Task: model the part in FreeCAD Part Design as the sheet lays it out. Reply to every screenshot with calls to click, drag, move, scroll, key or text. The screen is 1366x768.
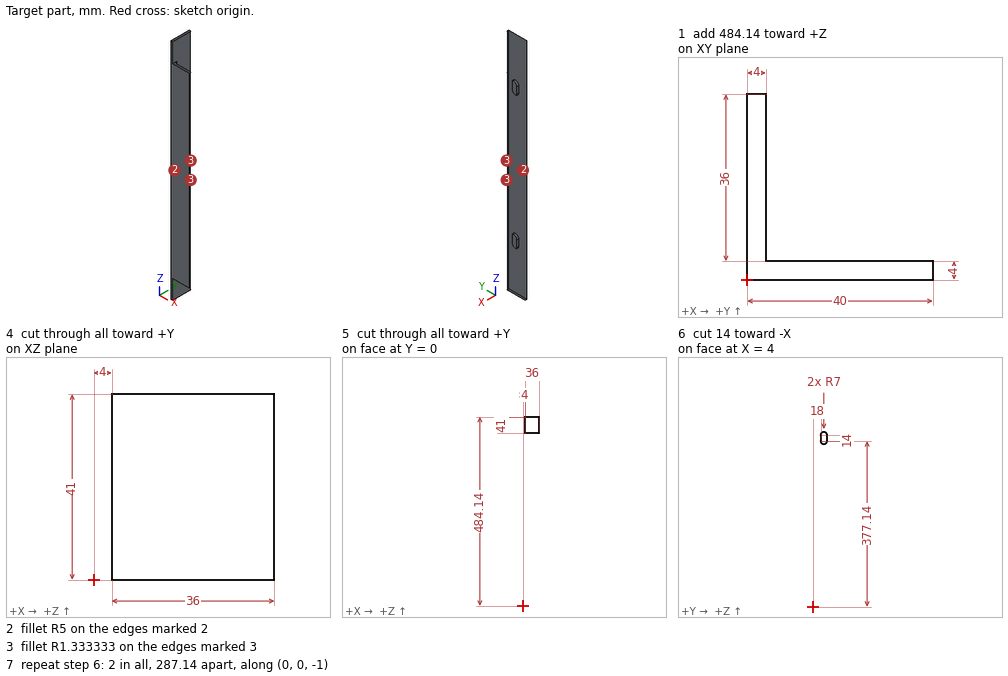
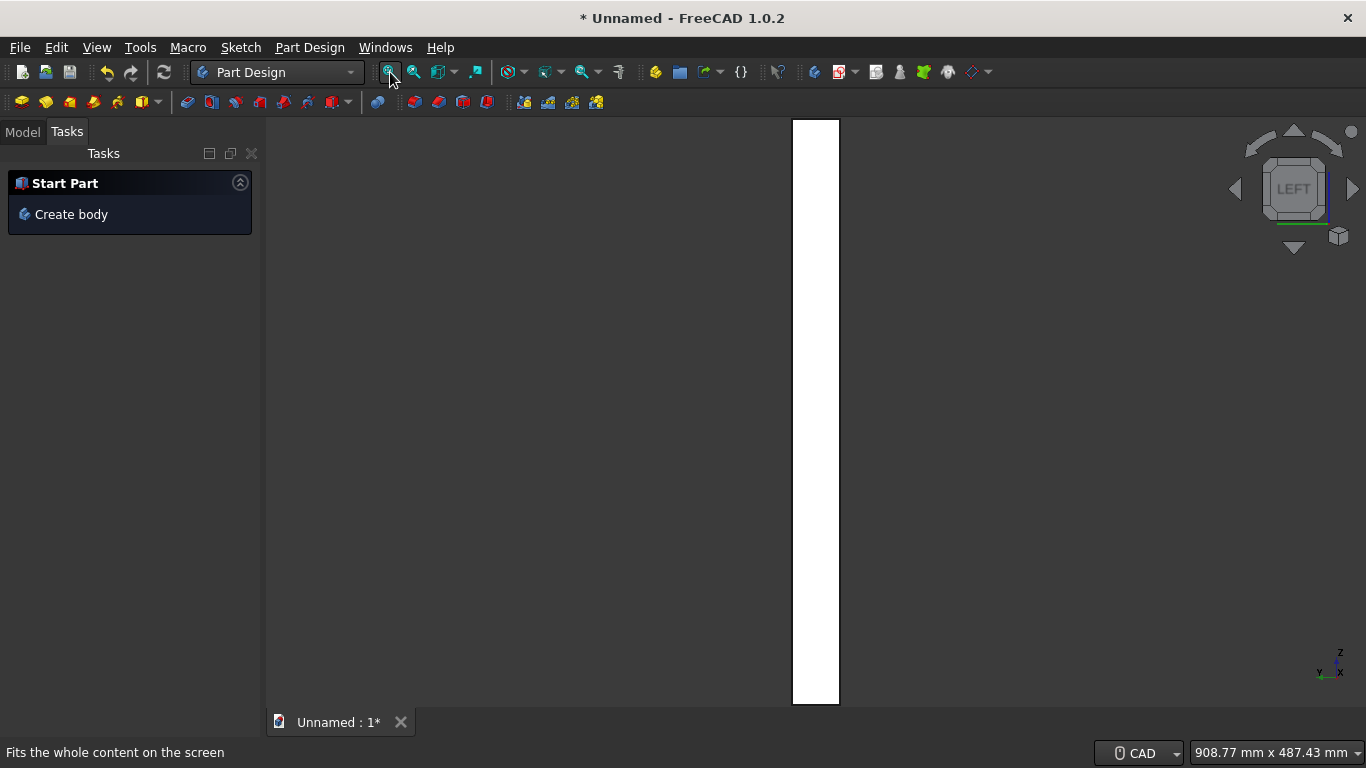
key(v)
key(3)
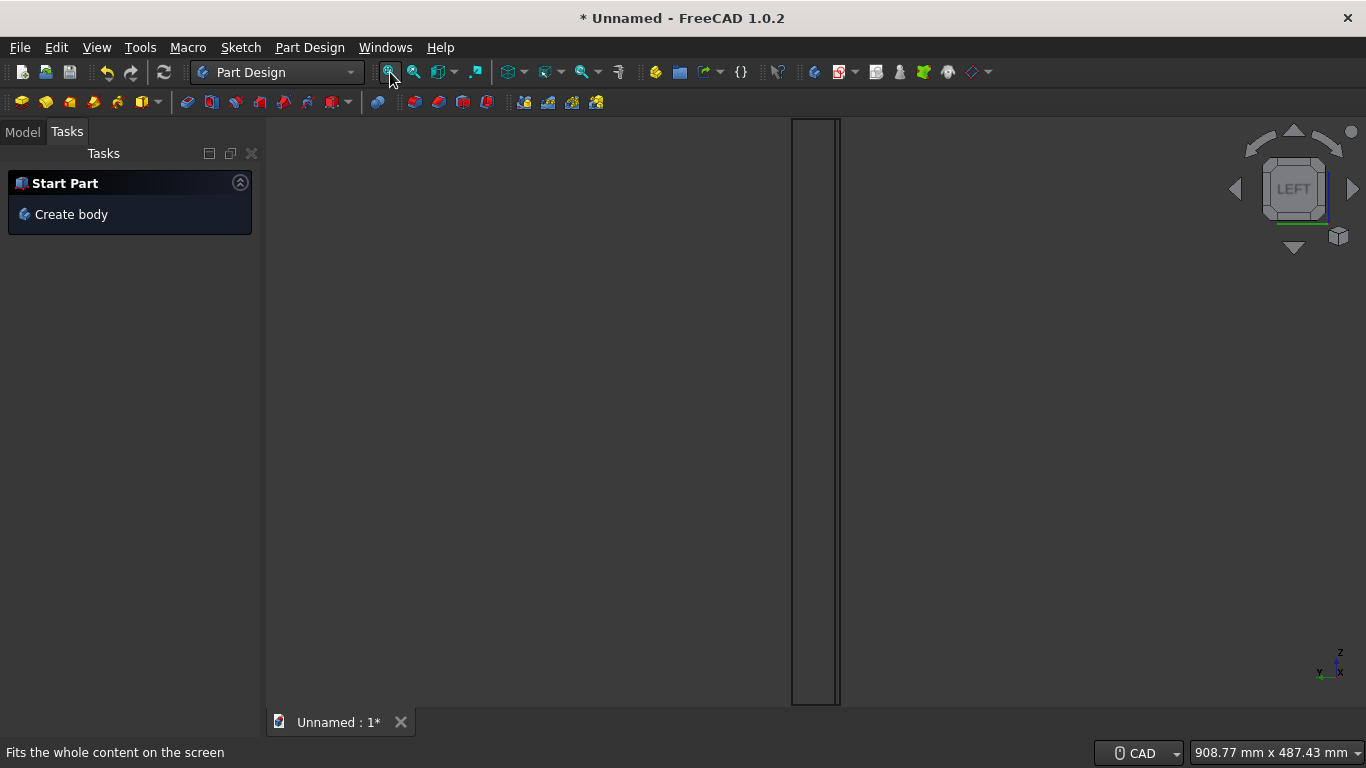
key(0)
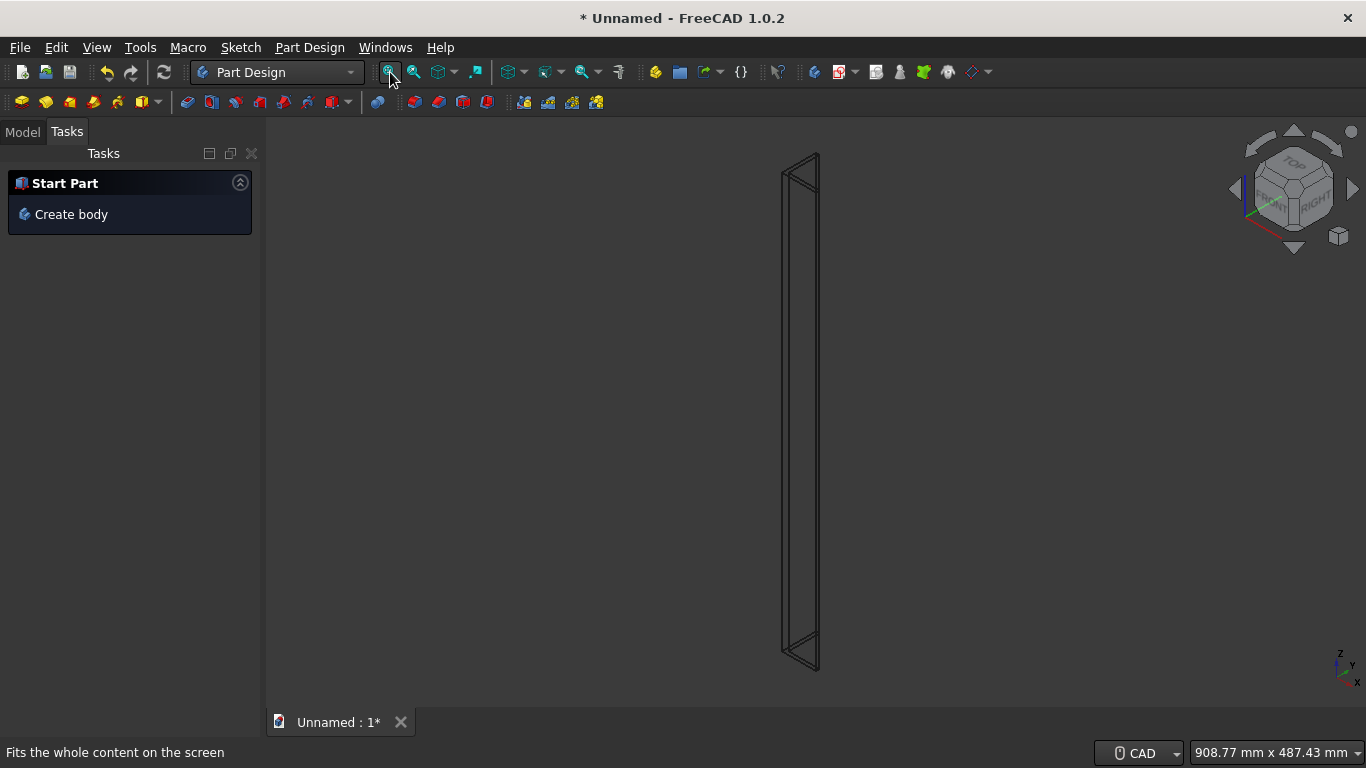
click(789, 411)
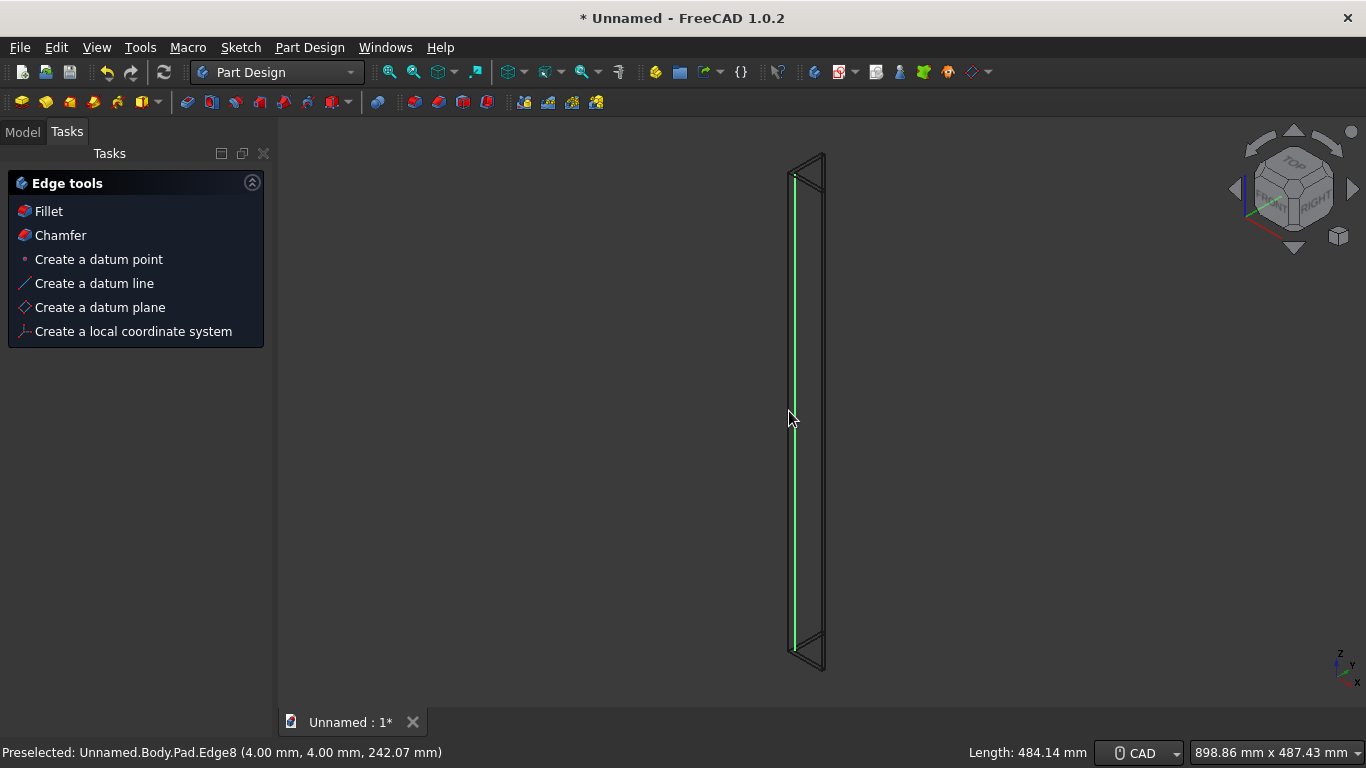
key(v)
key(1)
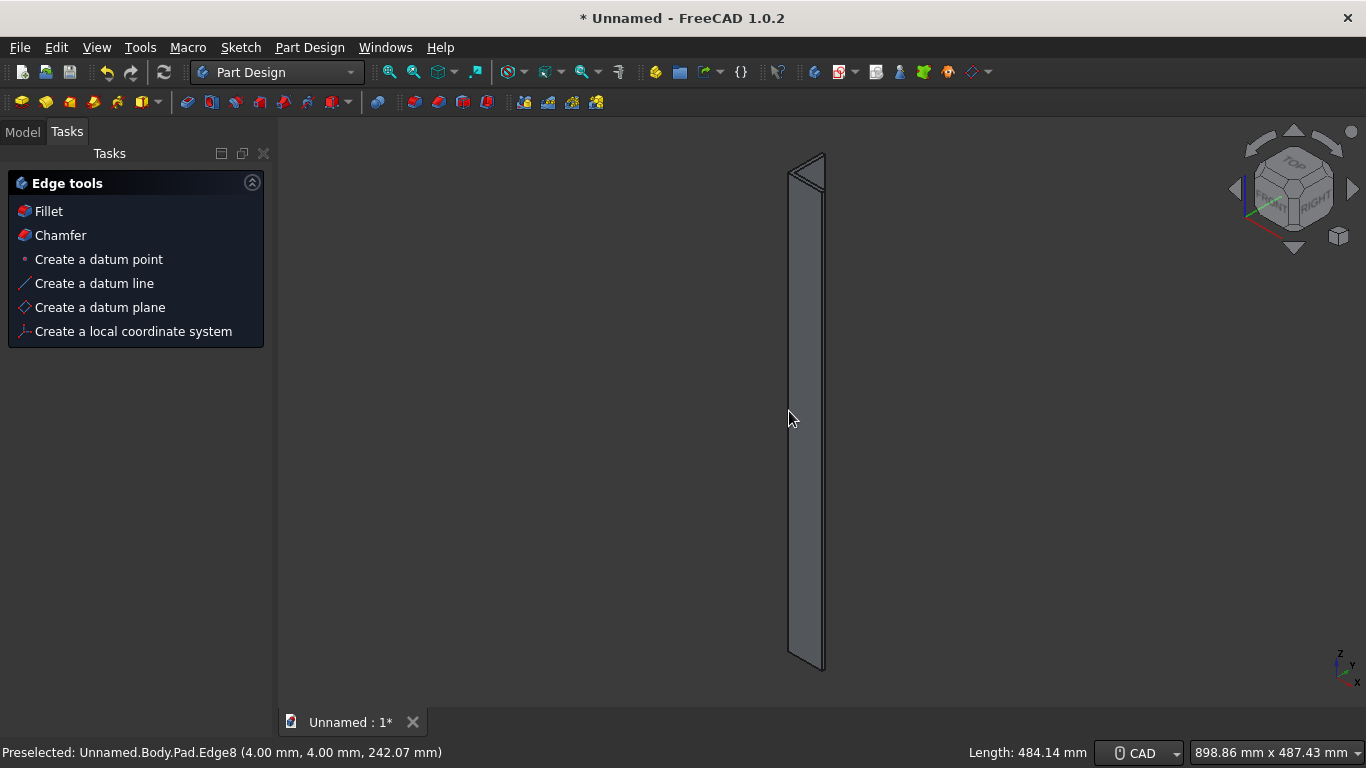
click(416, 102)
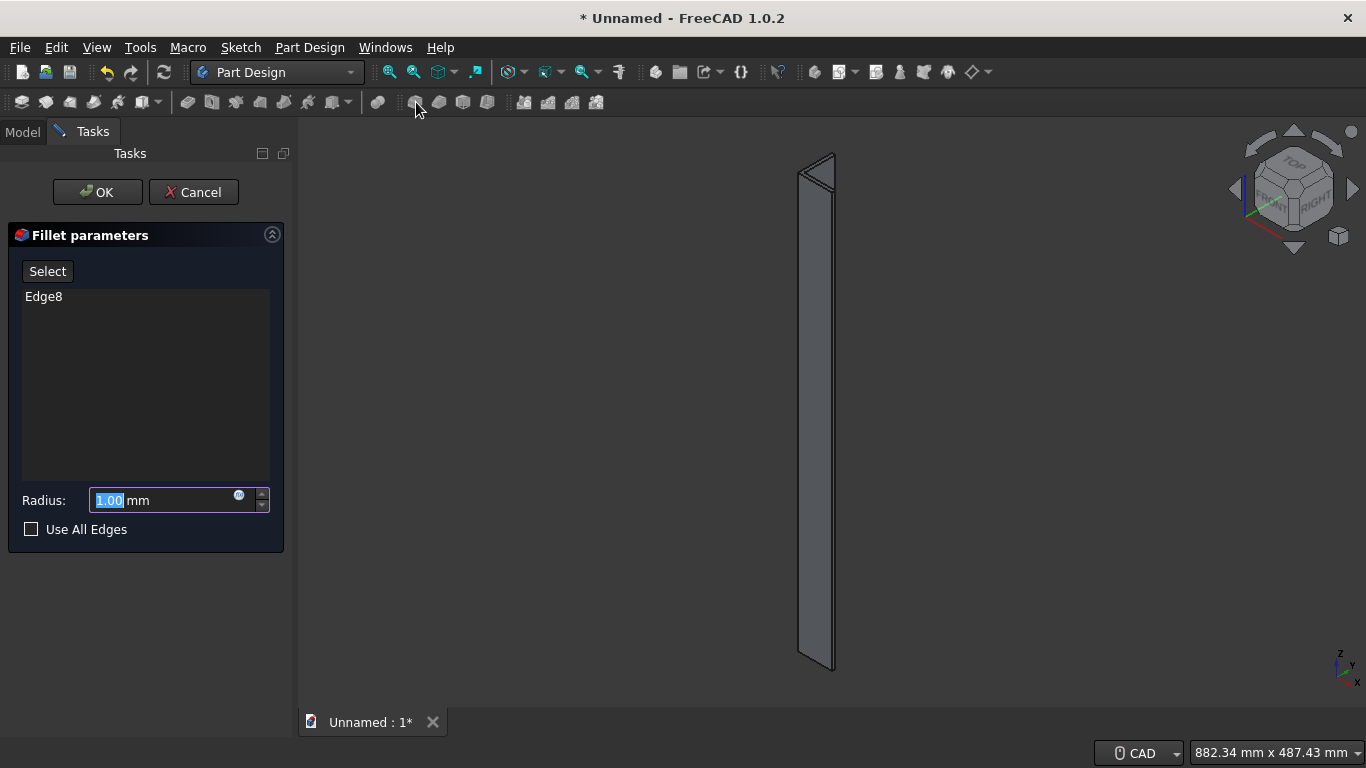
text(5)
key(Tab)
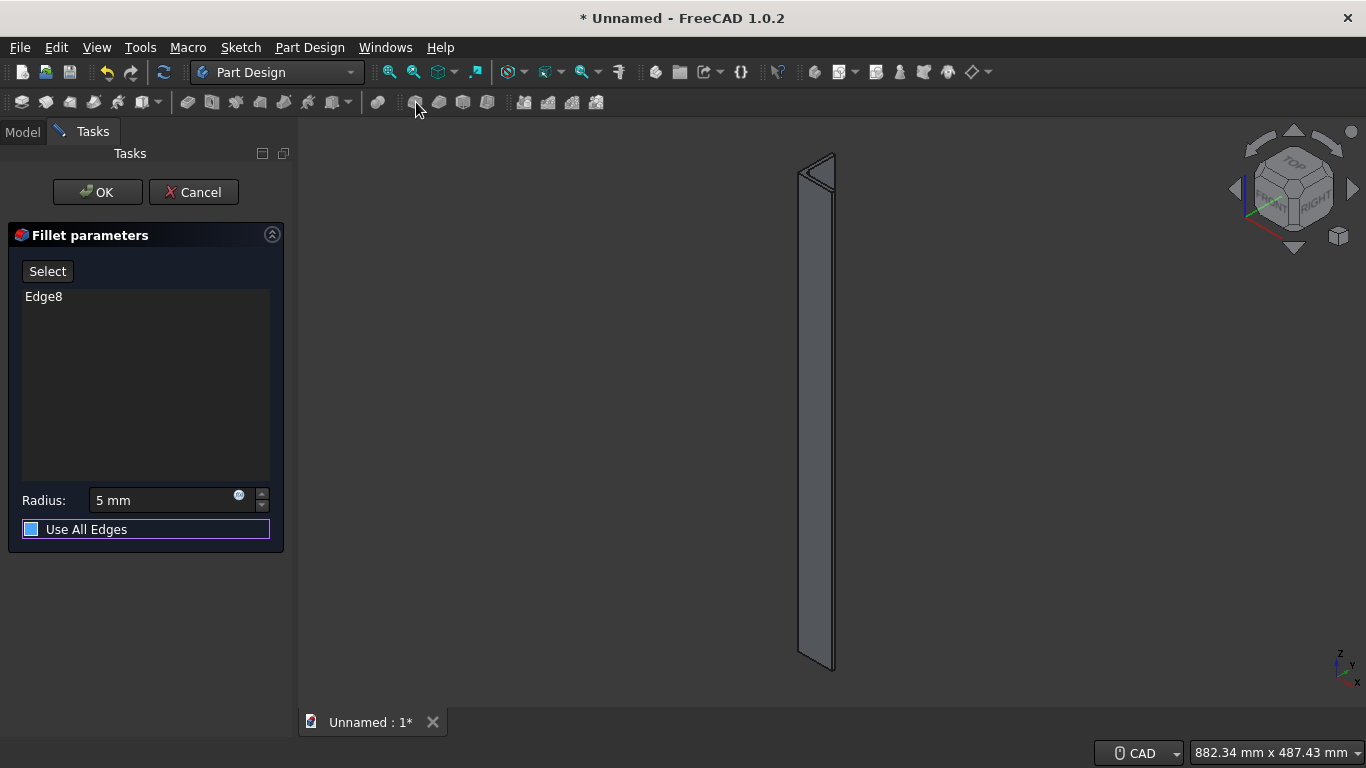
click(98, 192)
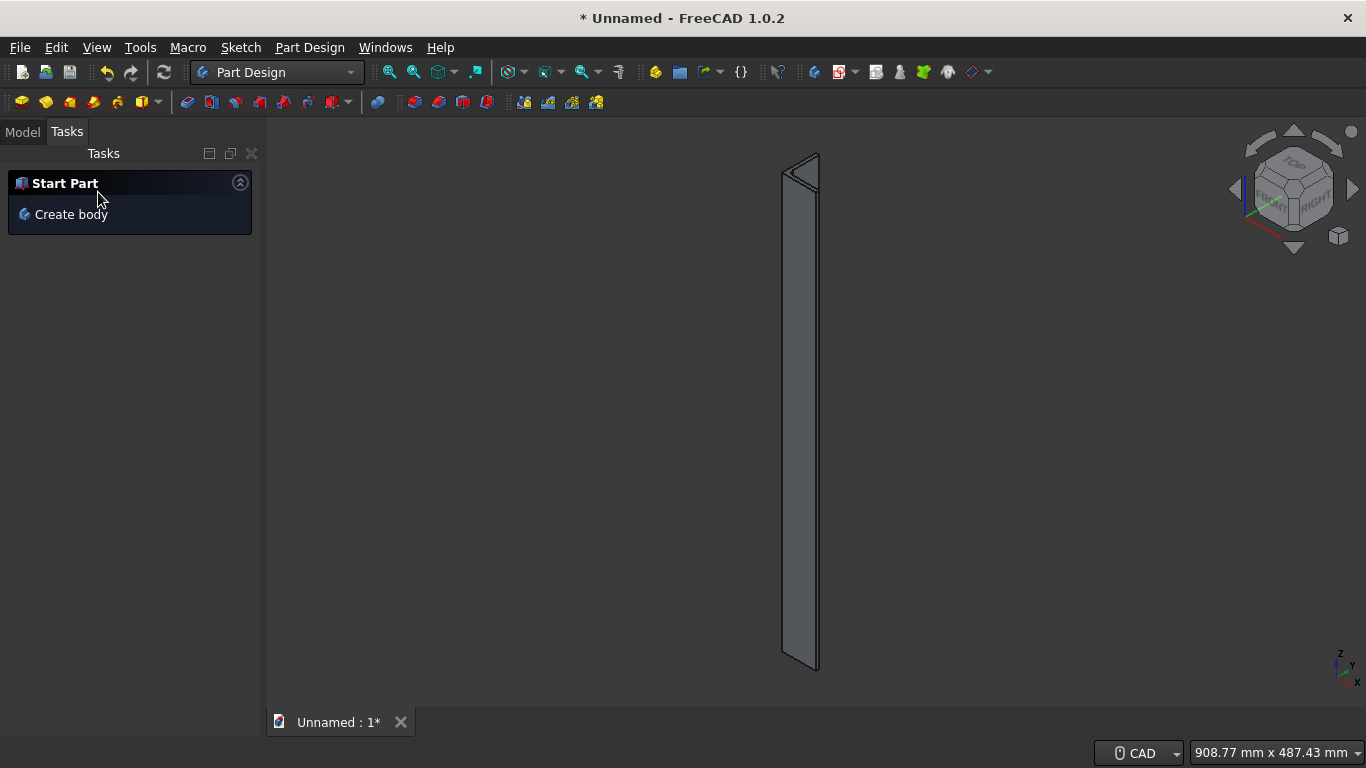
key(2)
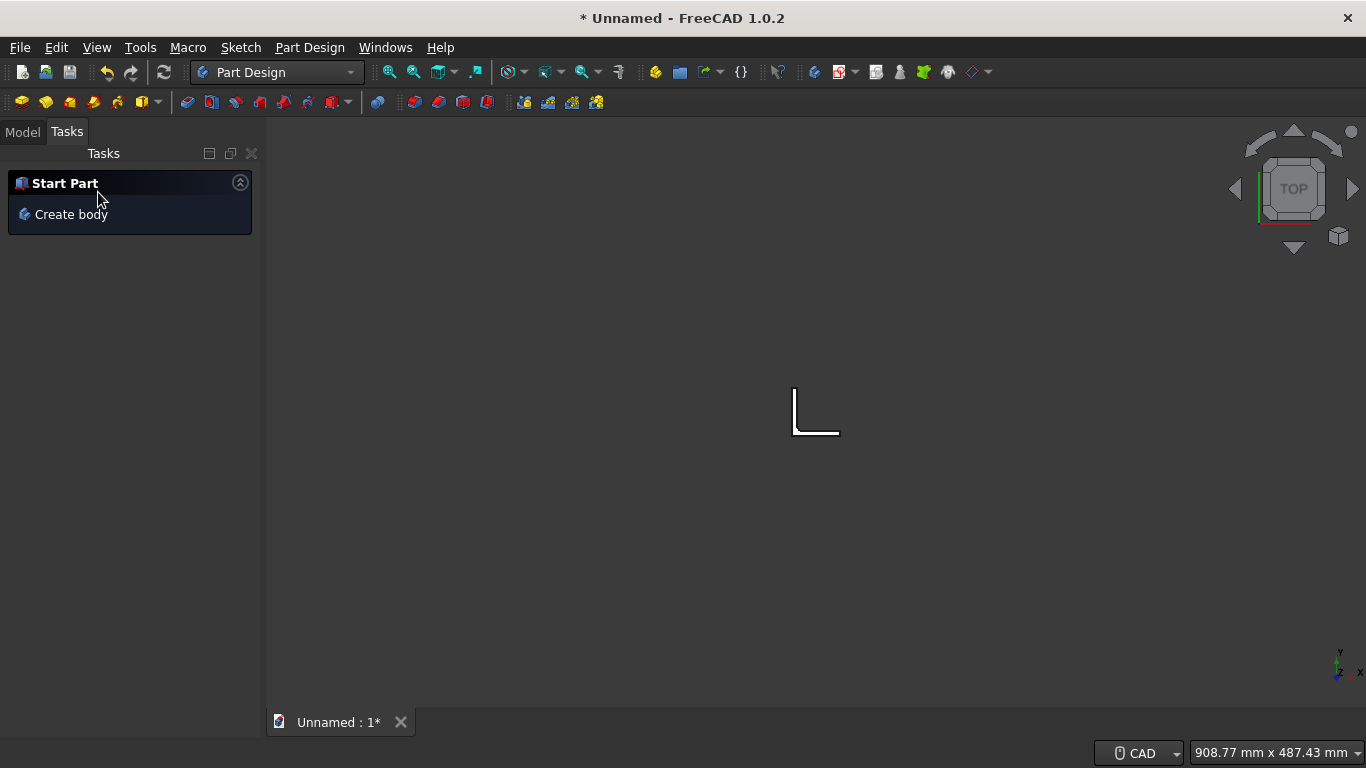
click(390, 72)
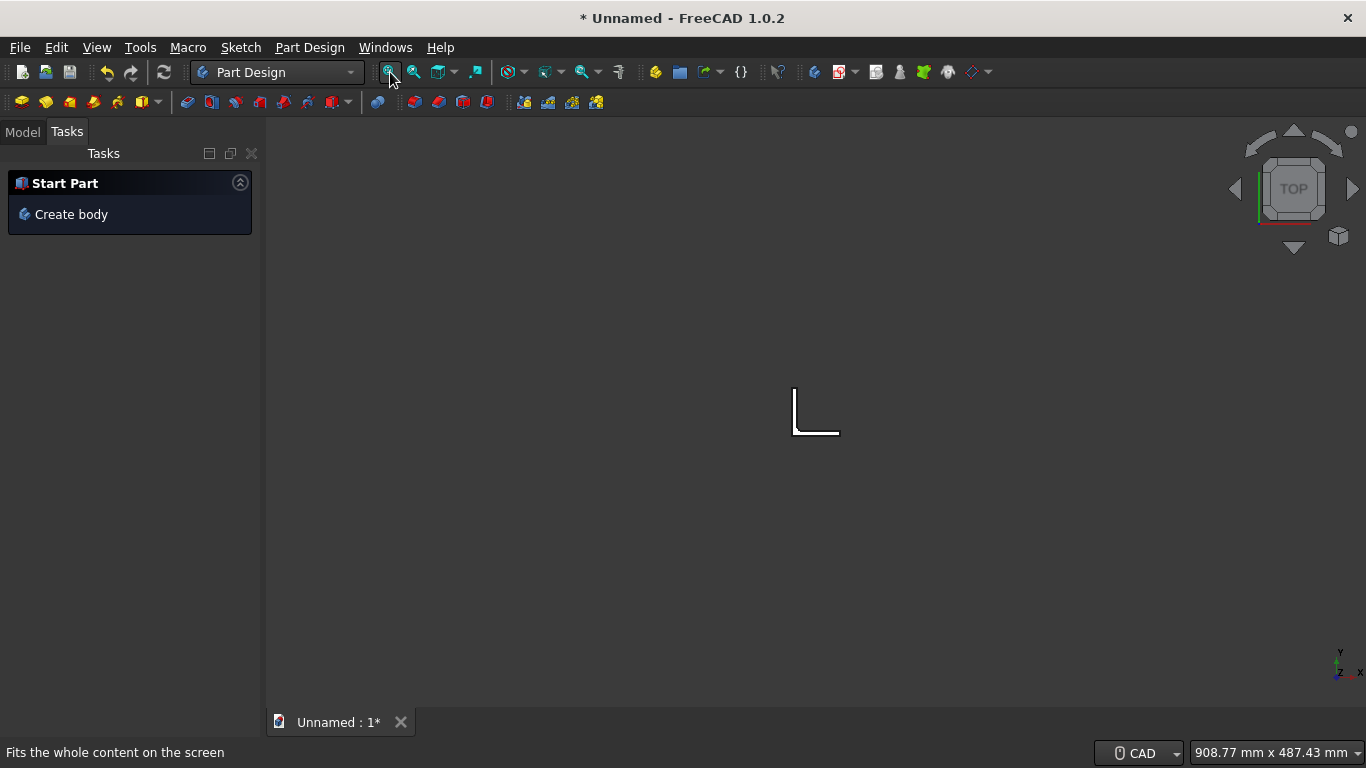
key(0)